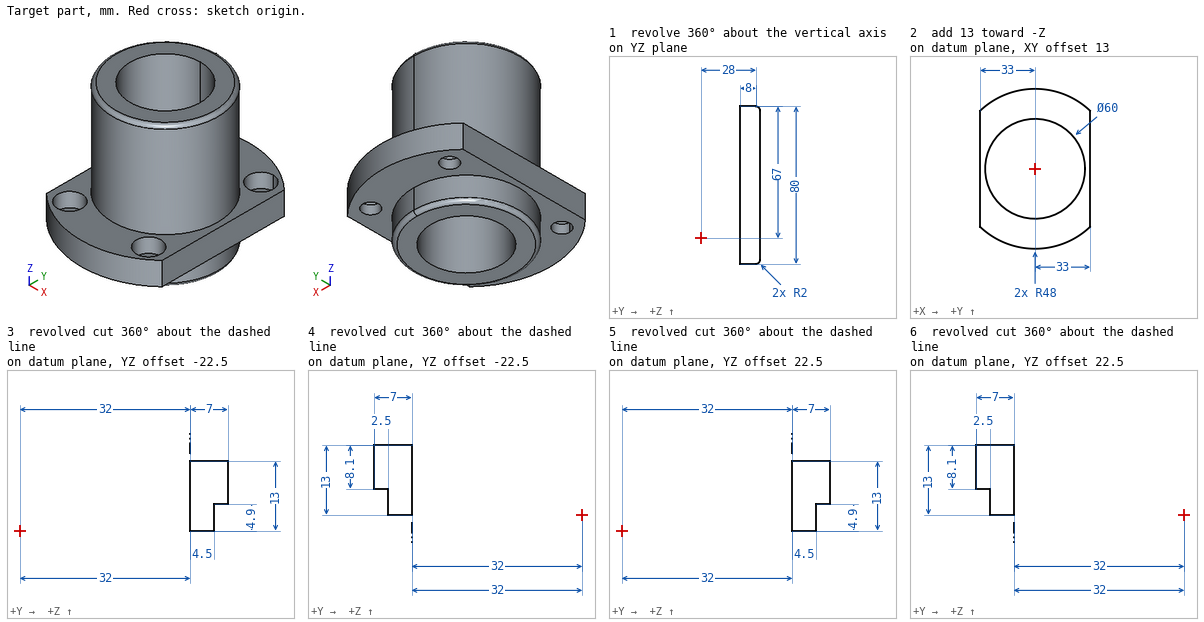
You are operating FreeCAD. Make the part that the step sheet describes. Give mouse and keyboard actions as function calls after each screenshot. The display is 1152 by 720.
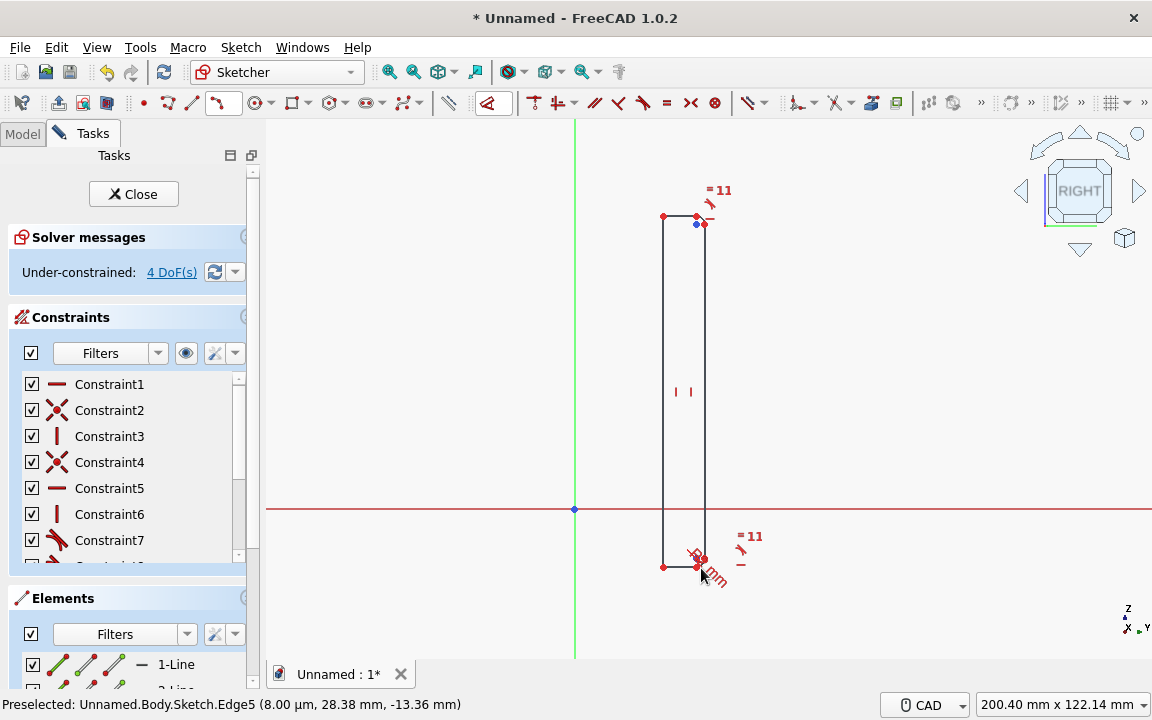
scroll(686, 216, up, 2)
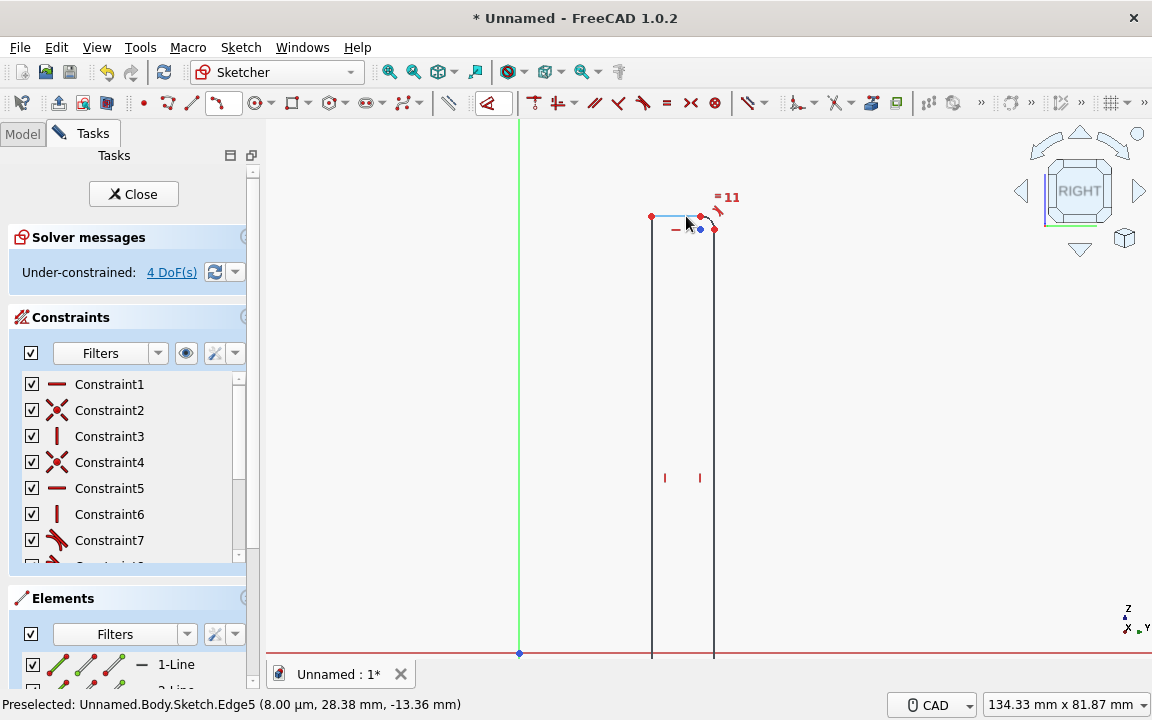
click(686, 216)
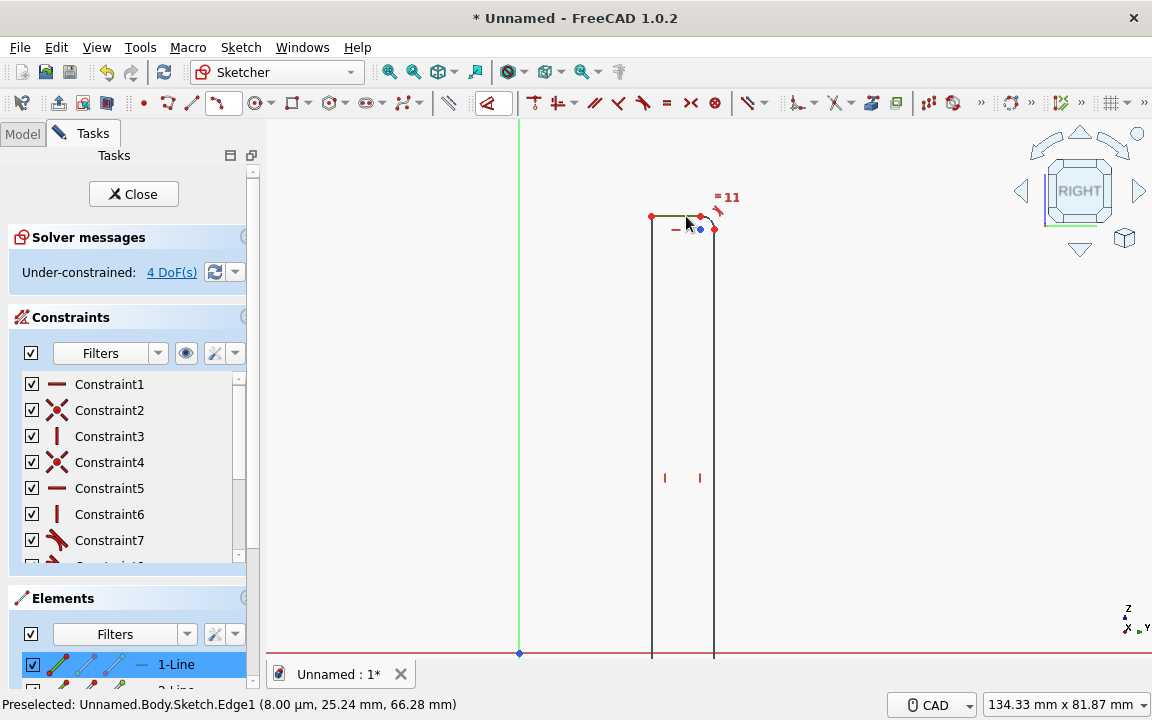
key(l)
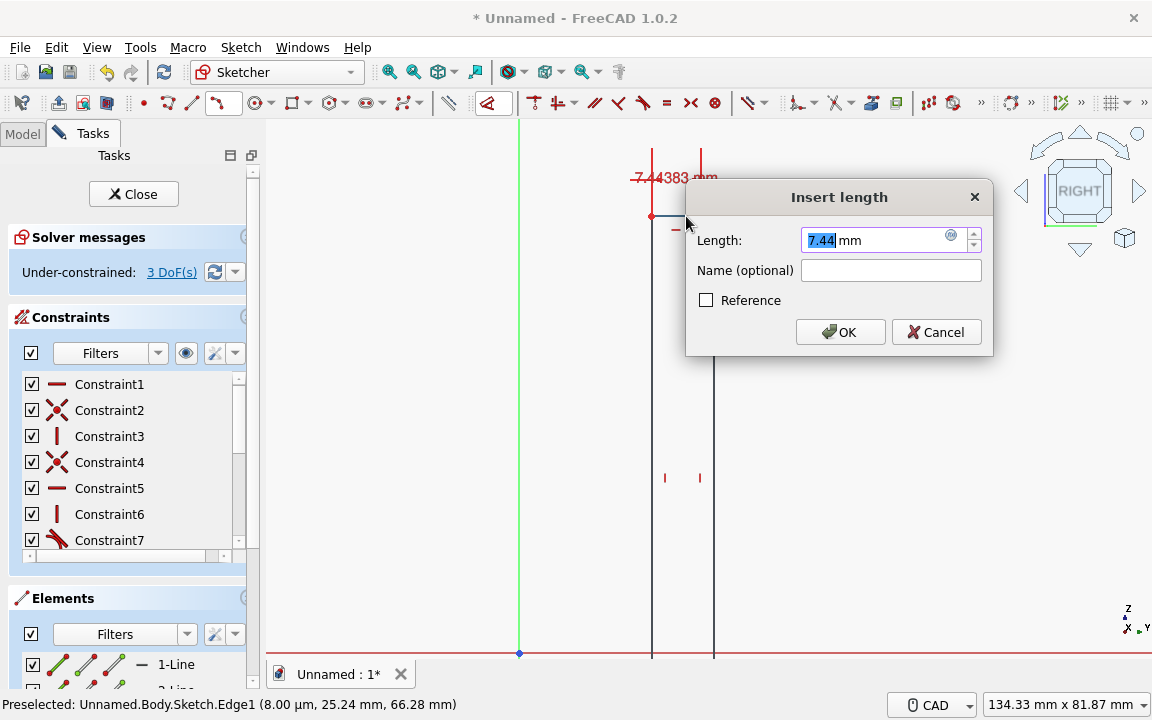
text(8)
key(Return)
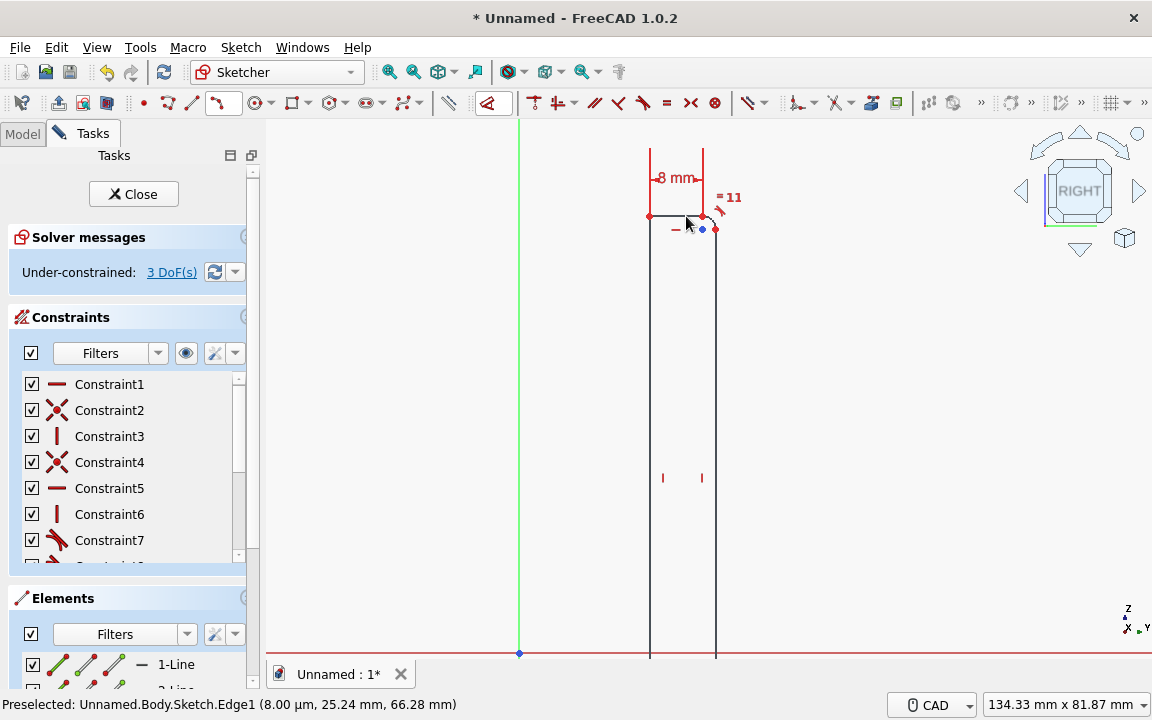
click(650, 373)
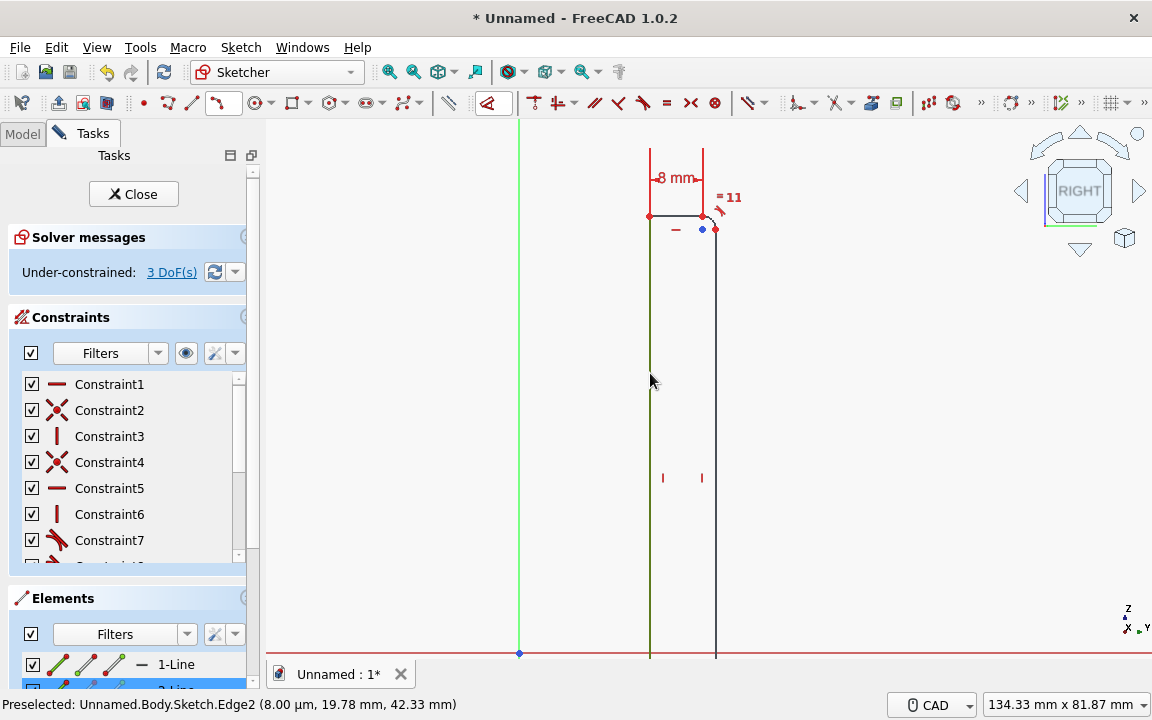
click(506, 104)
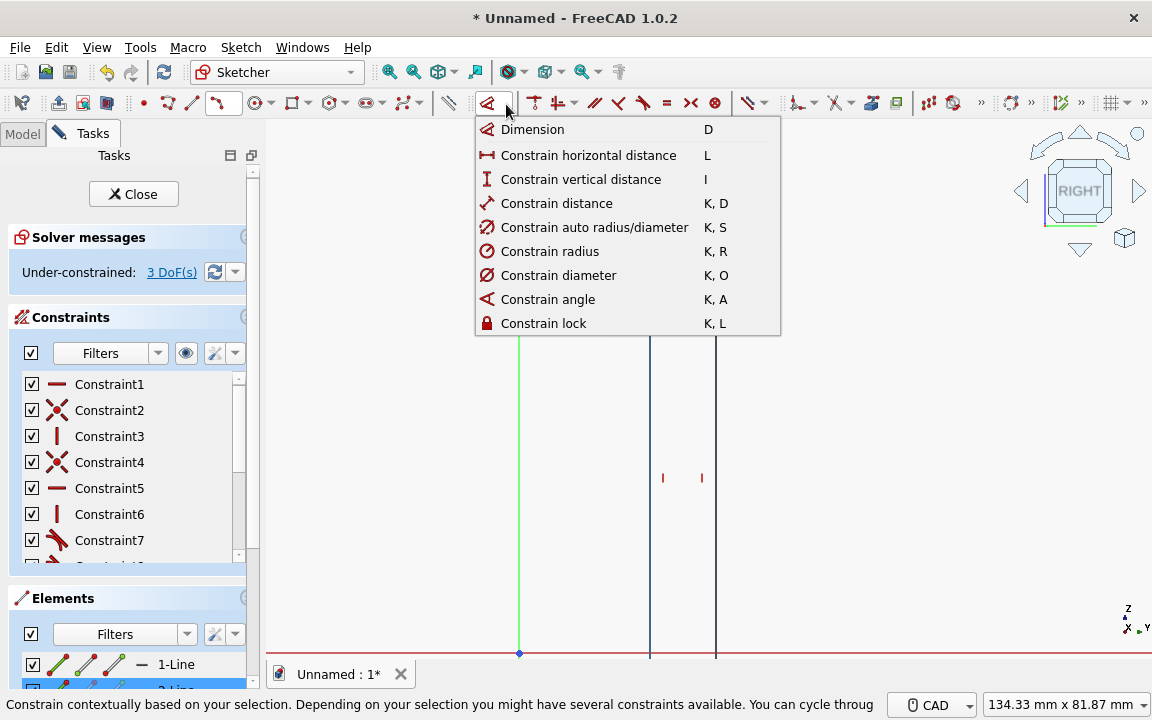
click(628, 179)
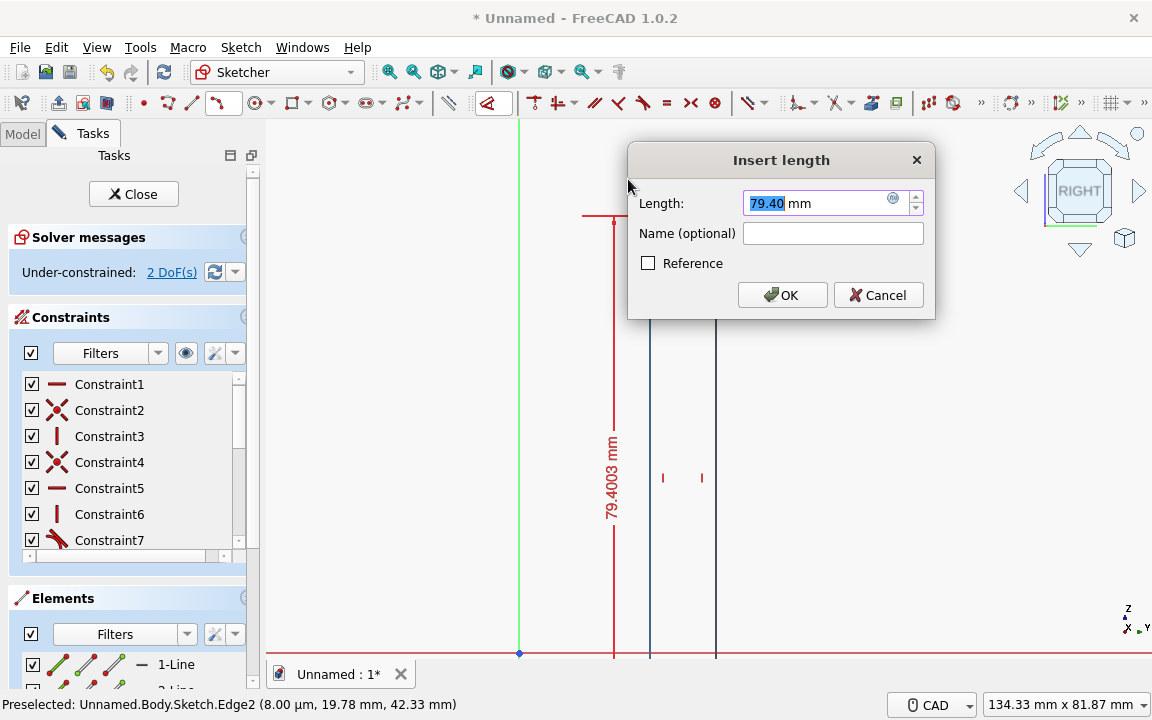
text(80)
key(Return)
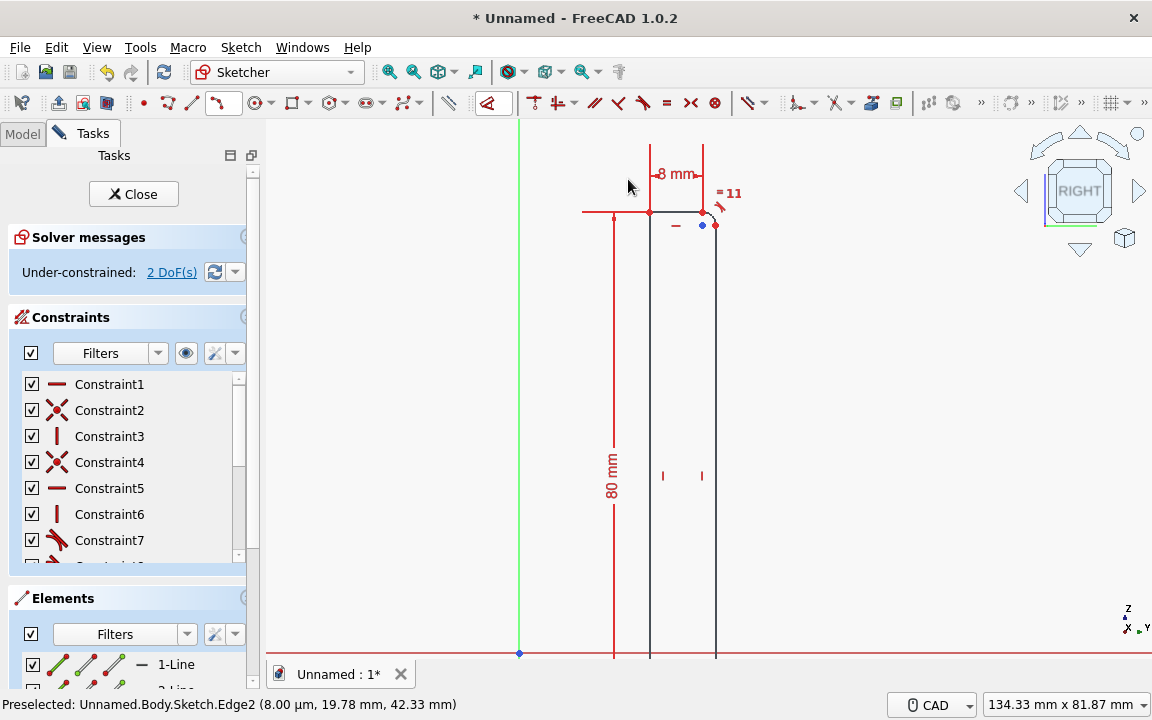
click(703, 212)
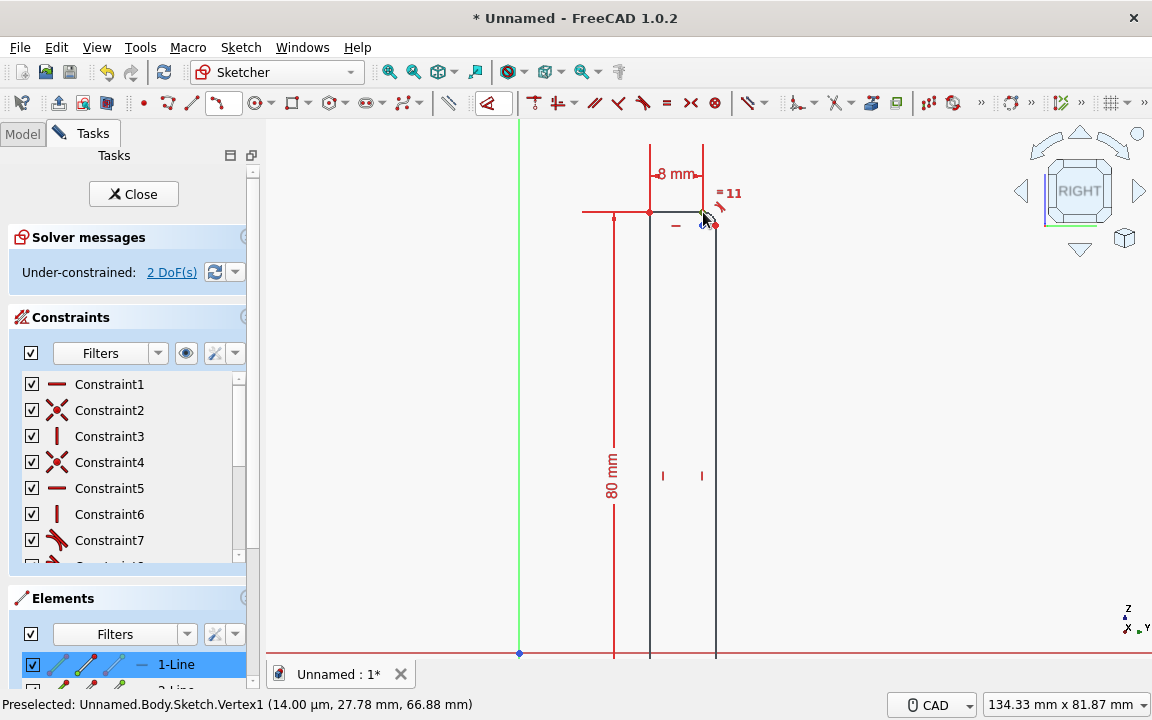
click(506, 104)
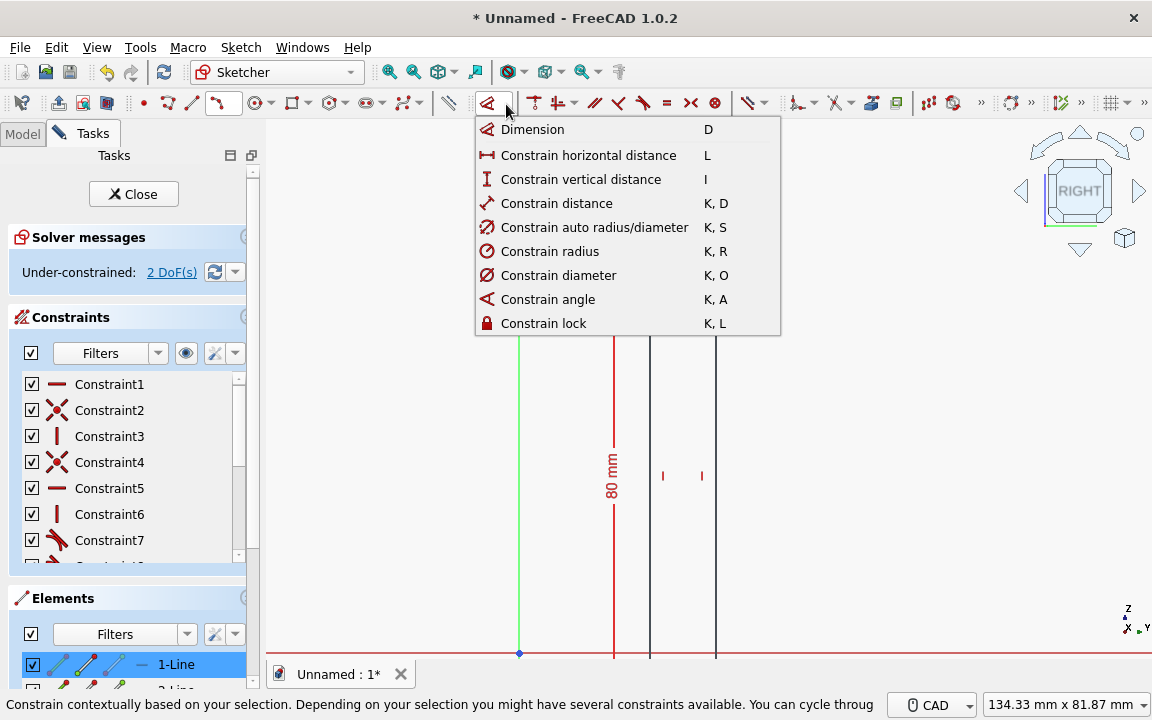
click(628, 155)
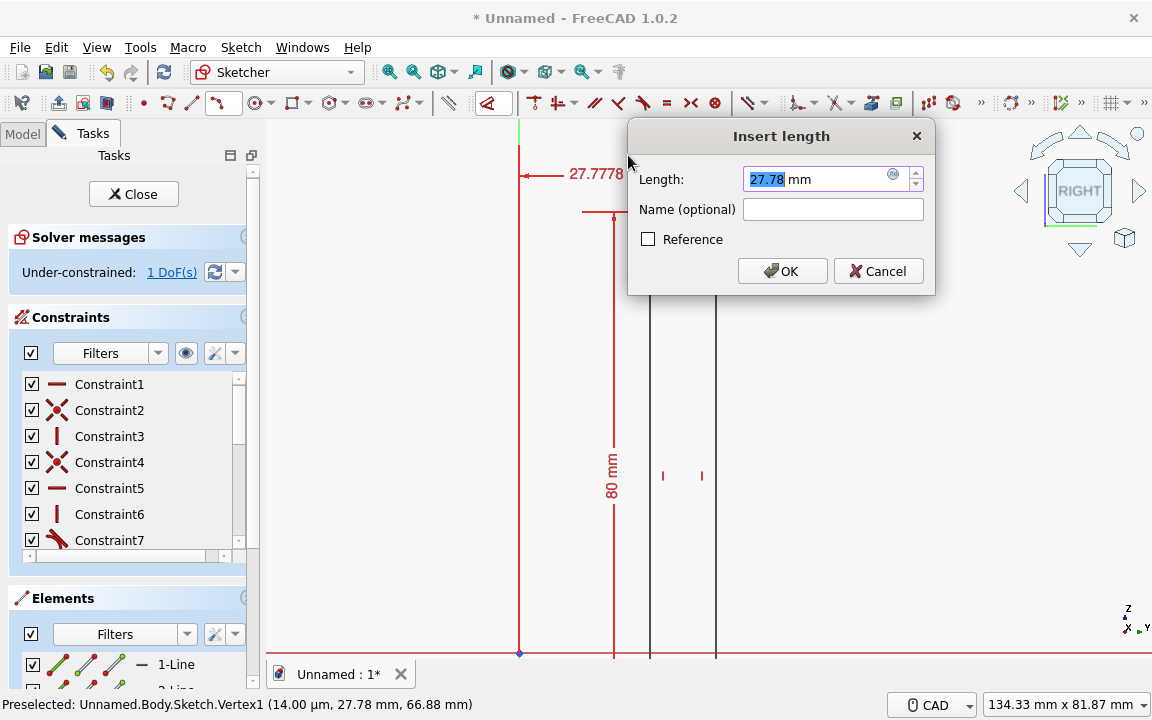
text(28)
key(Return)